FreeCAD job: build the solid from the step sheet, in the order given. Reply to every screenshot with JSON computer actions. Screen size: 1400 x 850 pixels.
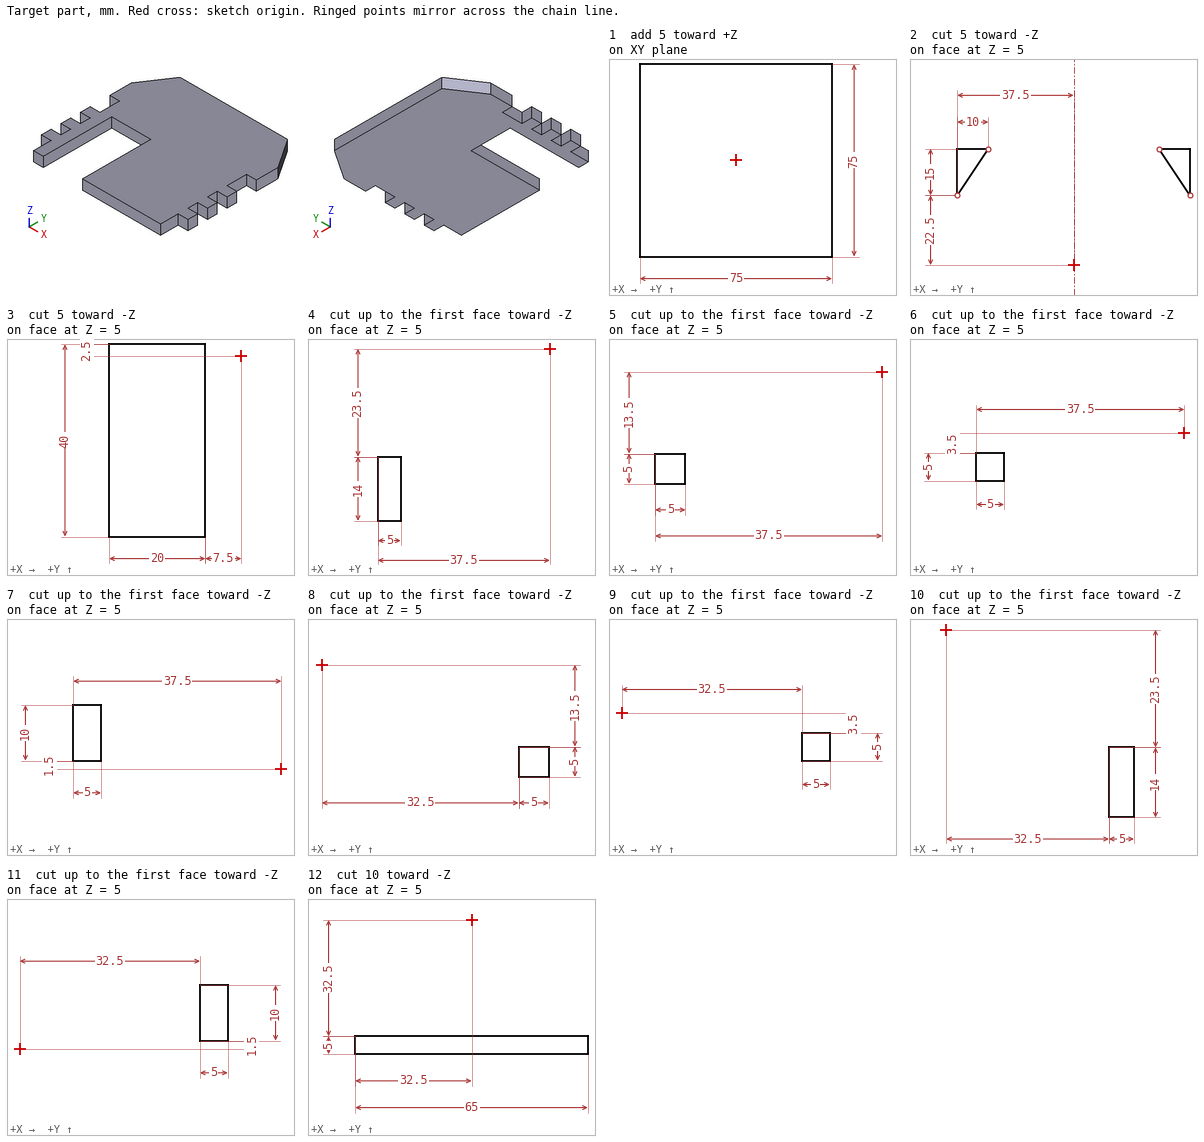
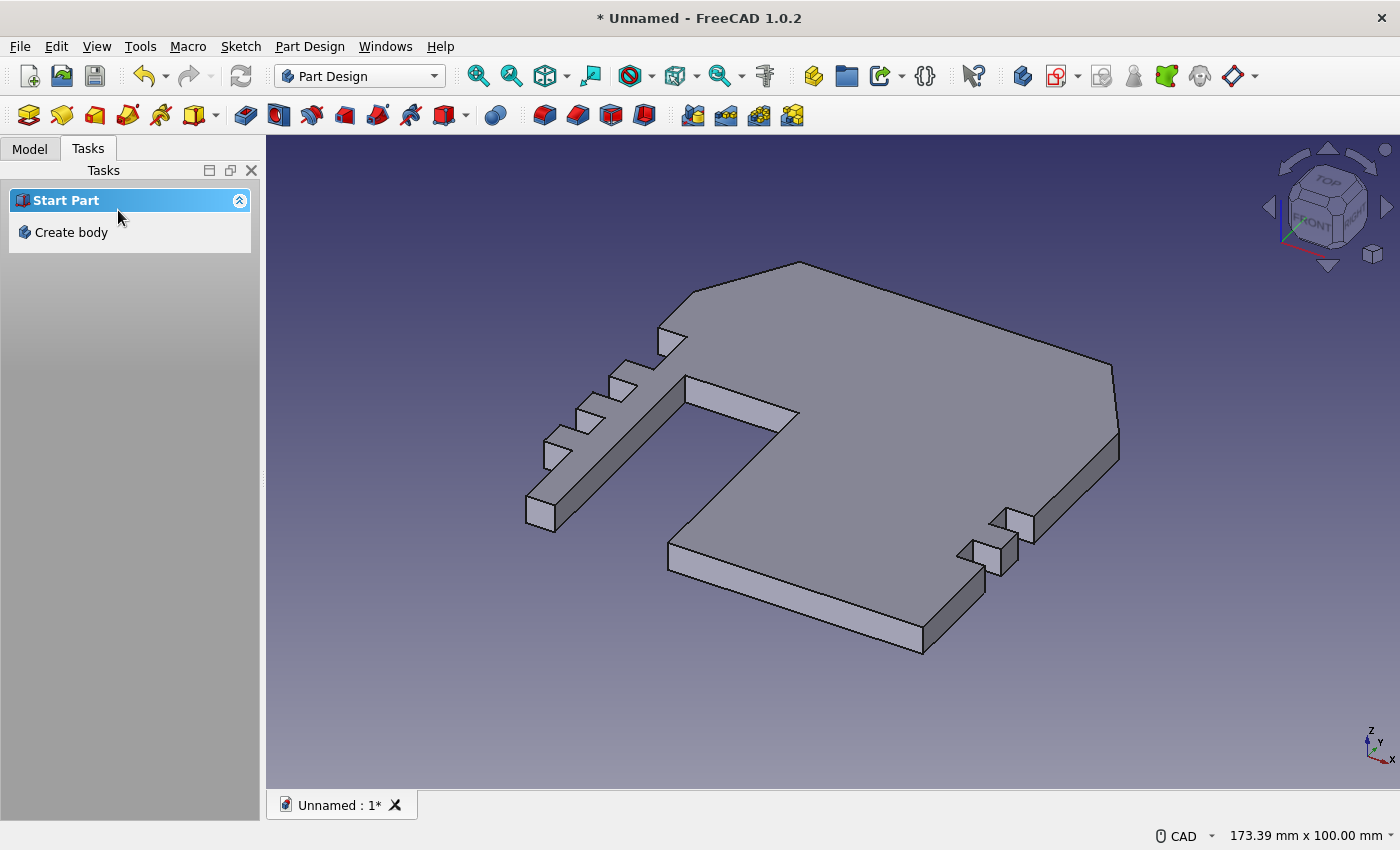
{"action": "left_click", "coordinate": [929, 420]}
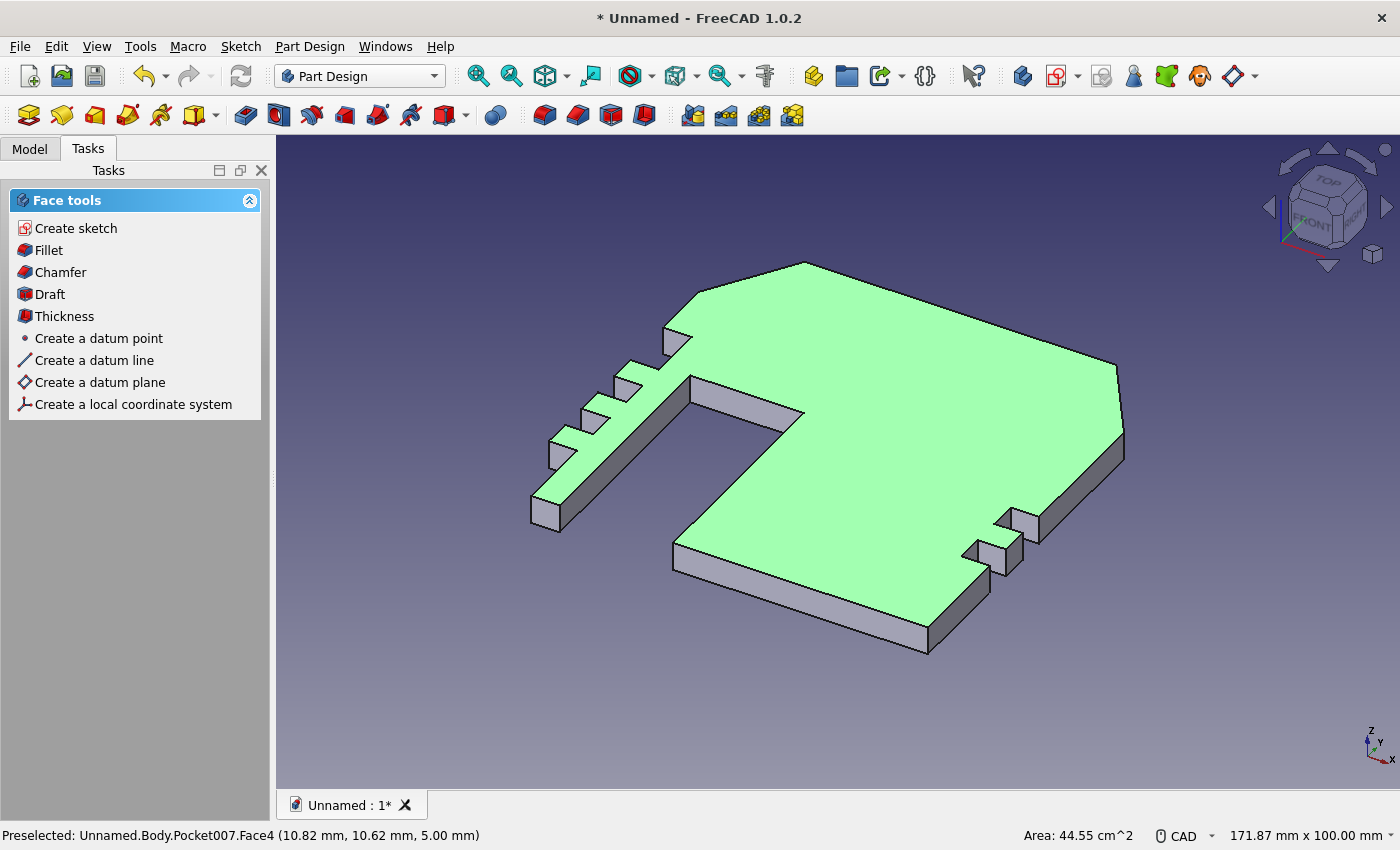
{"action": "left_click", "coordinate": [1056, 76]}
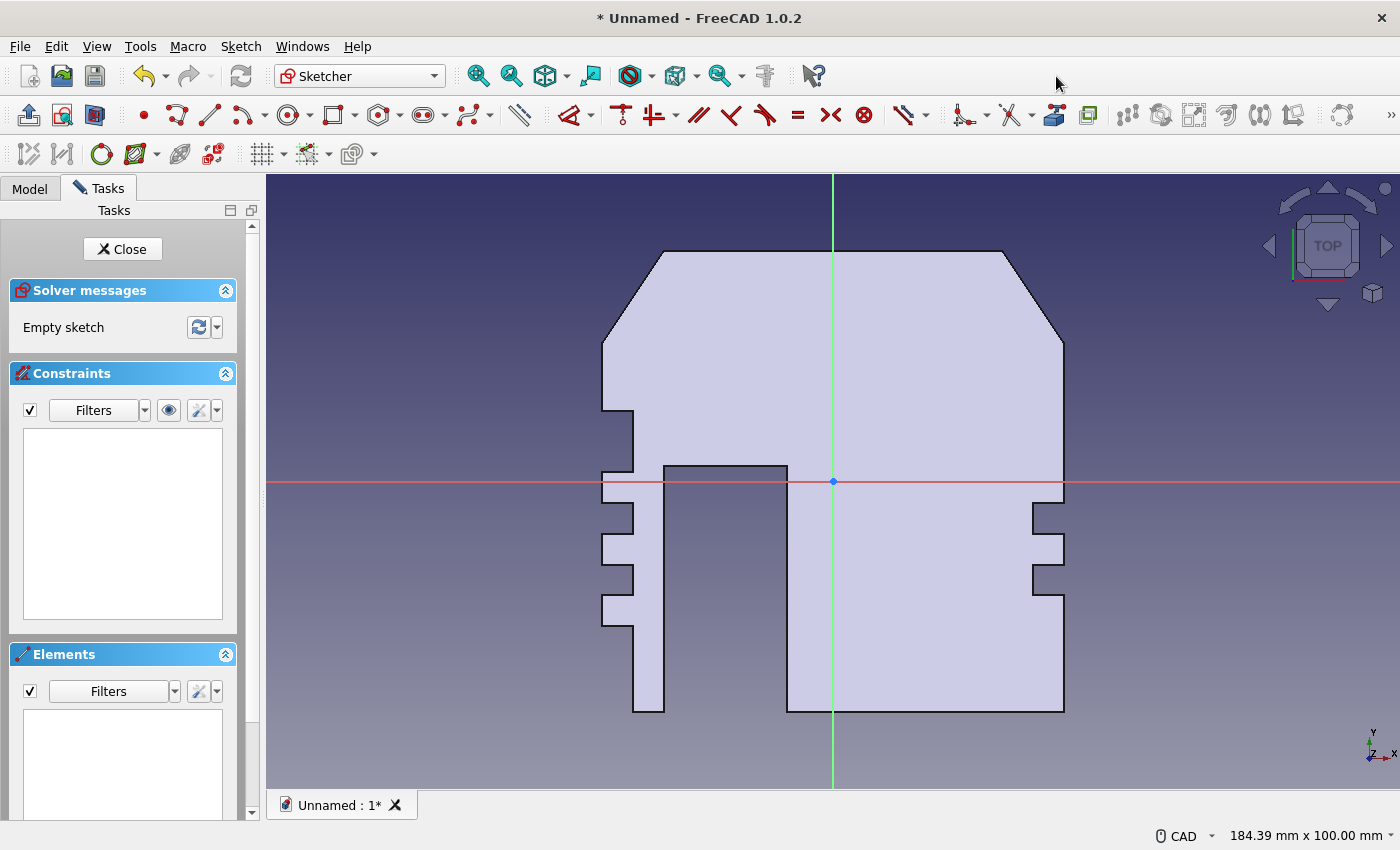
{"action": "scroll", "coordinate": [1120, 717], "scroll_direction": "up", "scroll_amount": 8}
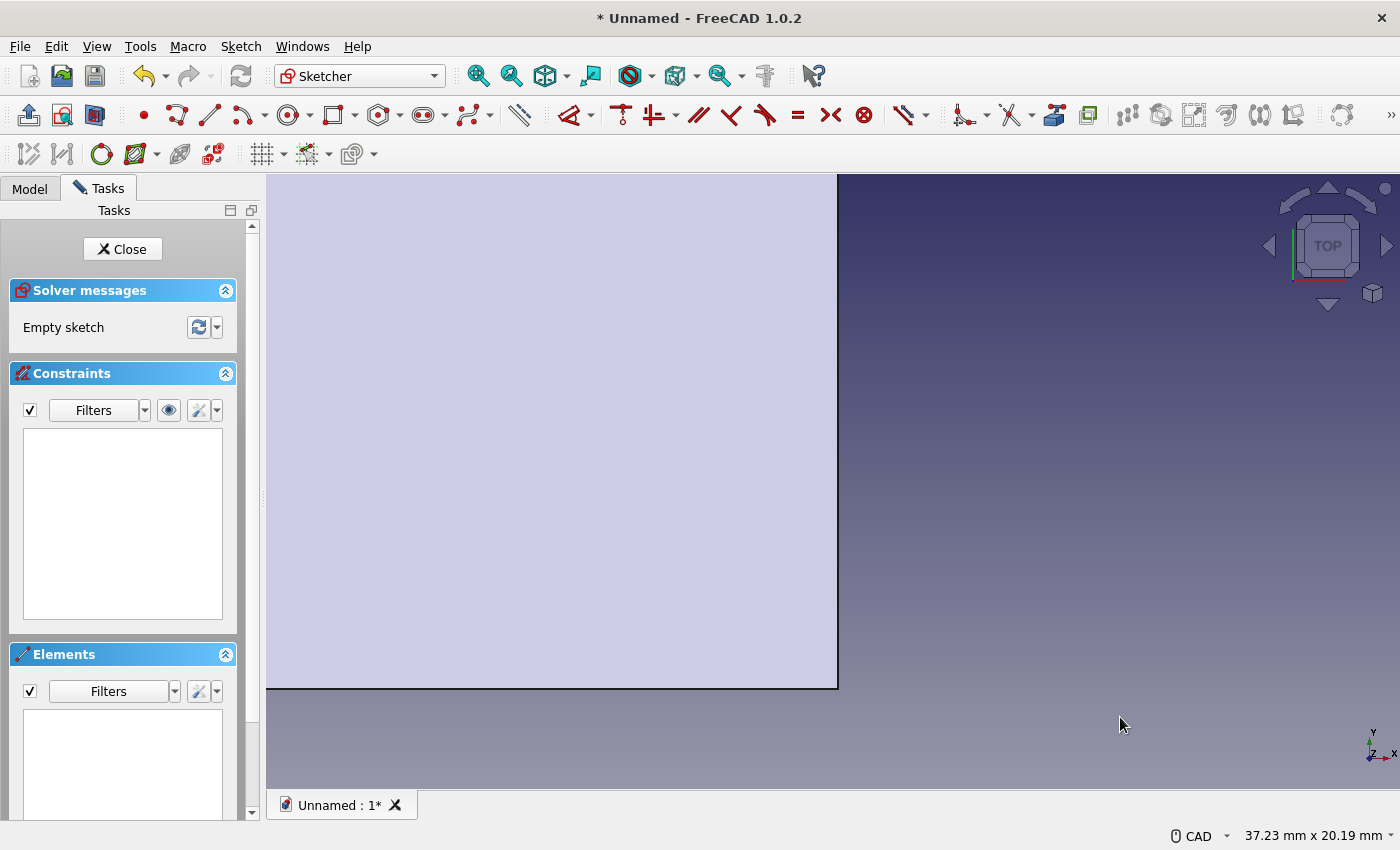
{"action": "left_click", "coordinate": [332, 116]}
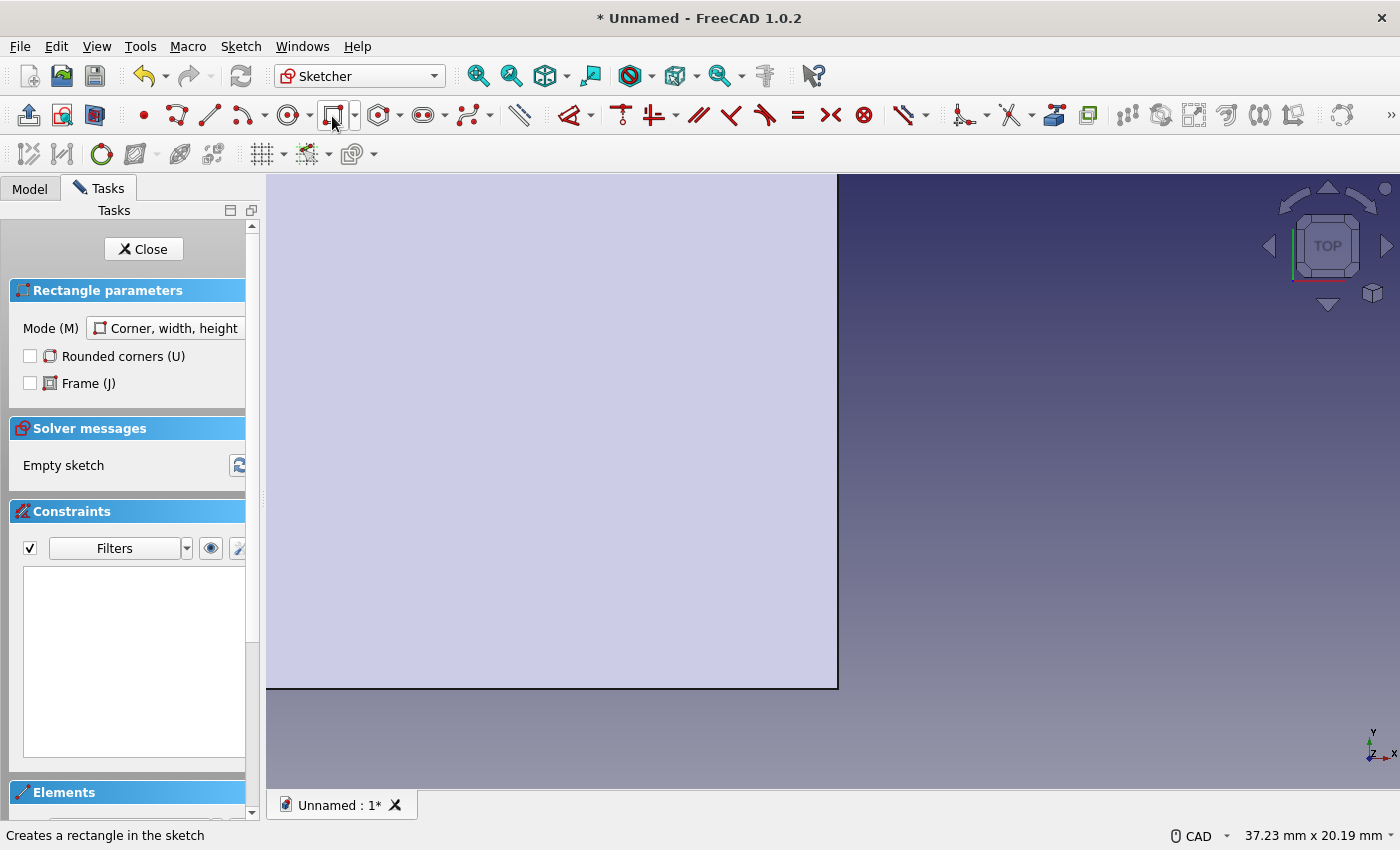
{"action": "left_click", "coordinate": [685, 263]}
{"action": "left_click", "coordinate": [838, 689]}
{"action": "key", "text": "Escape"}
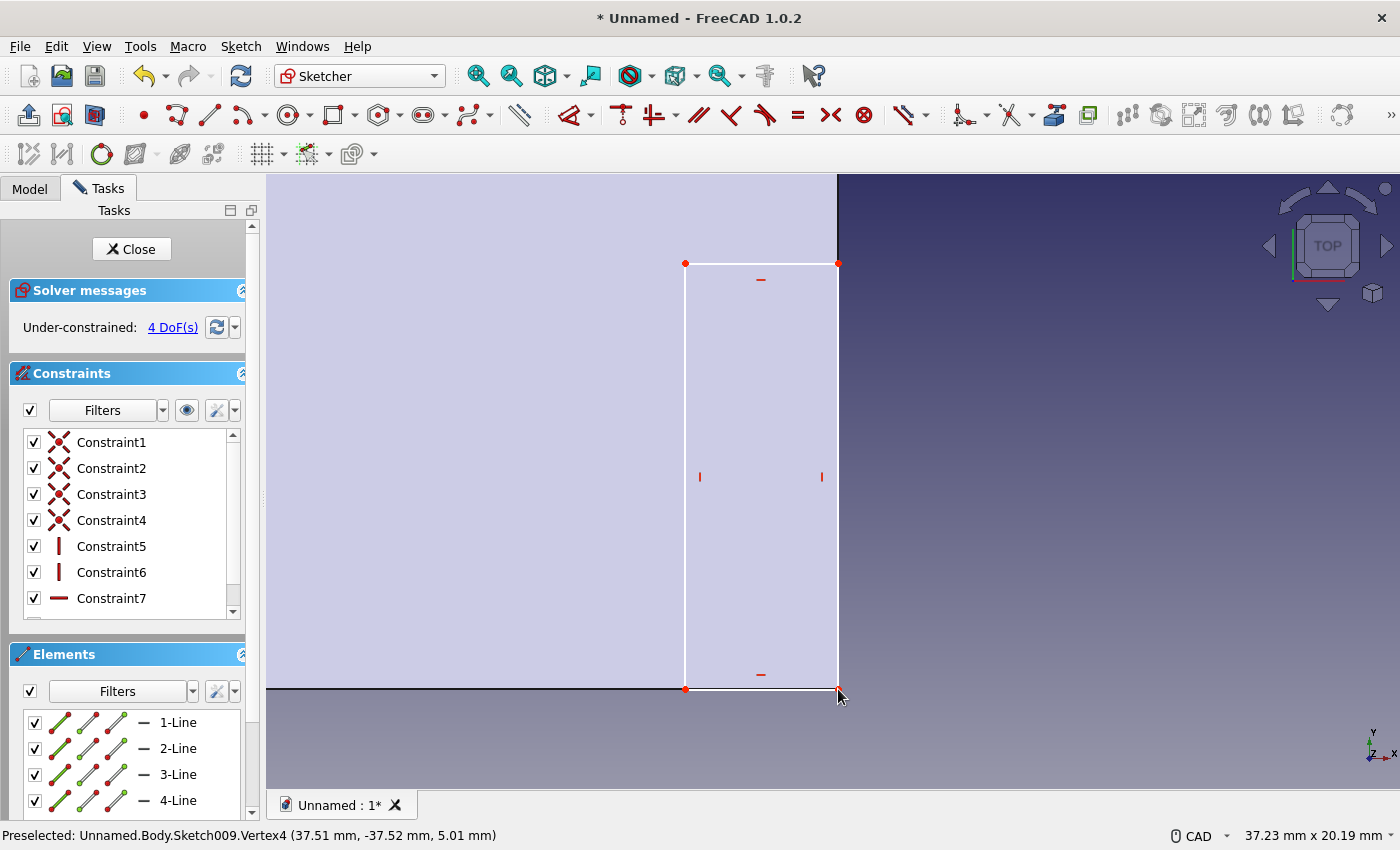
{"action": "key", "text": "d"}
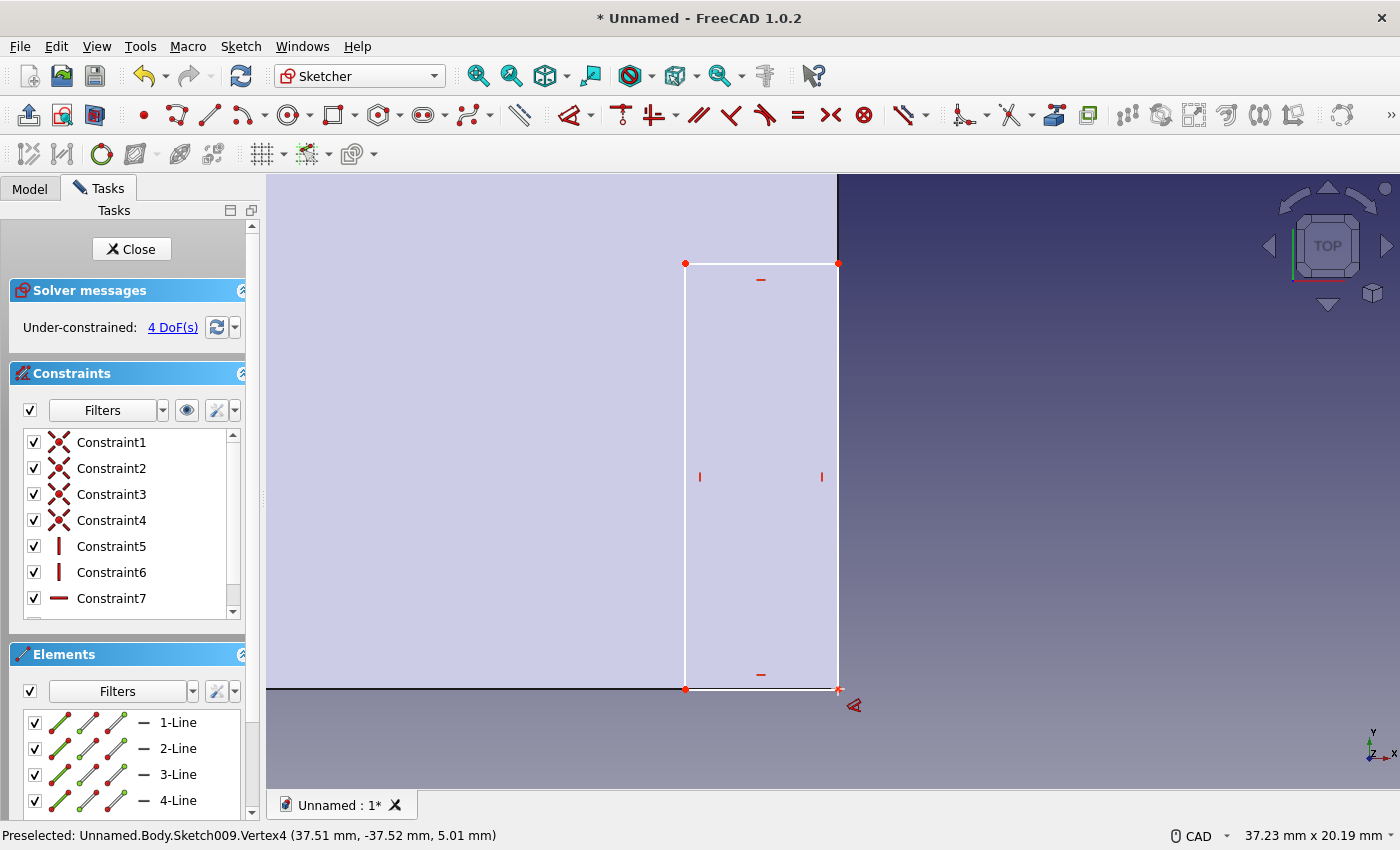
{"action": "left_click", "coordinate": [731, 690]}
{"action": "left_click", "coordinate": [762, 724]}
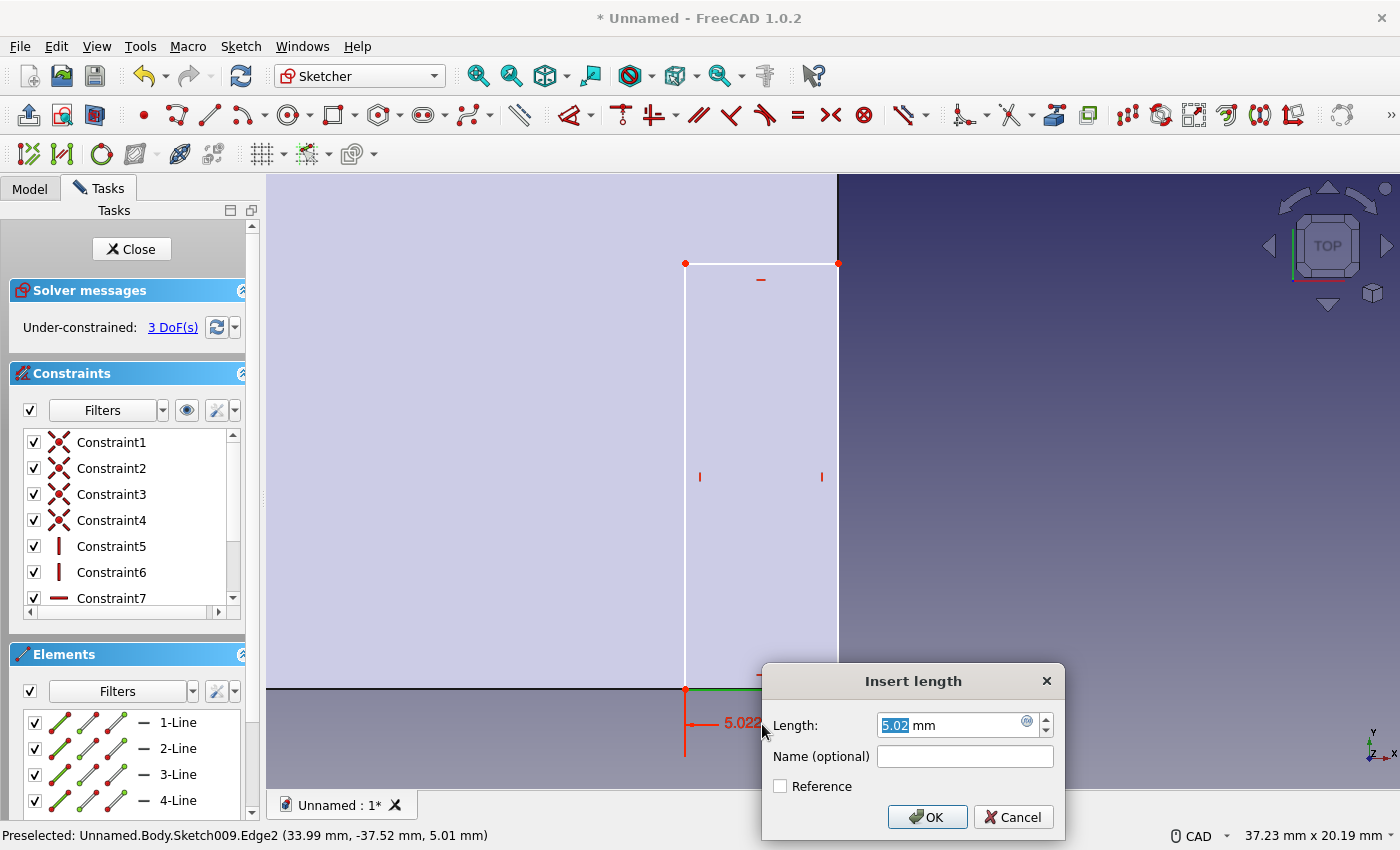
{"action": "type", "text": "5"}
{"action": "key", "text": "Return"}